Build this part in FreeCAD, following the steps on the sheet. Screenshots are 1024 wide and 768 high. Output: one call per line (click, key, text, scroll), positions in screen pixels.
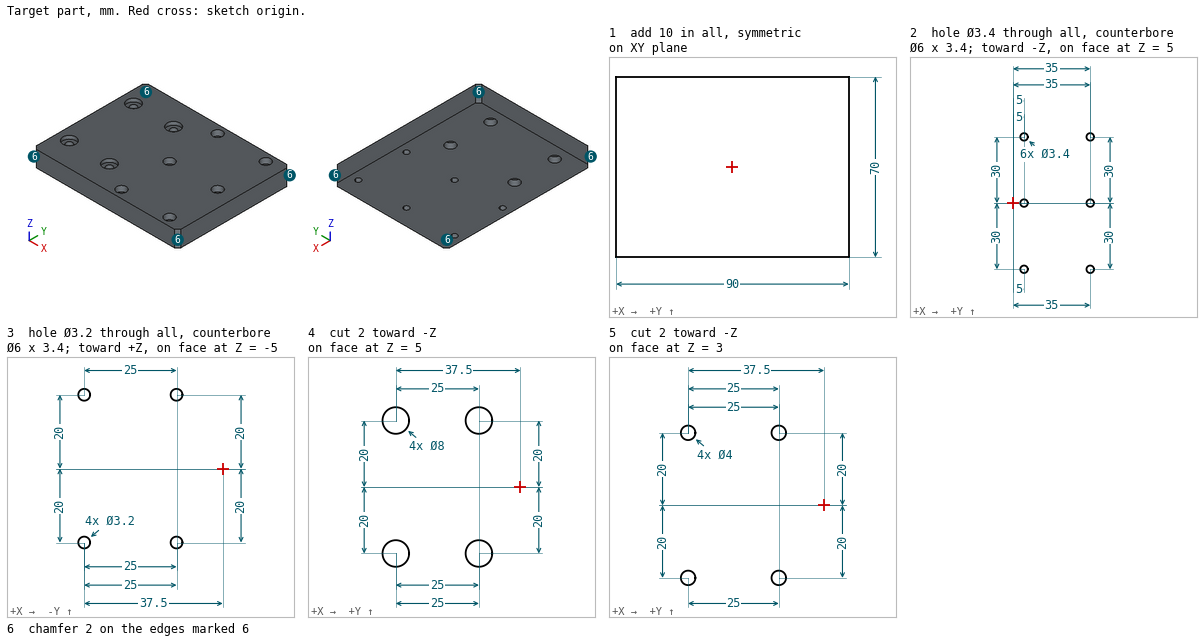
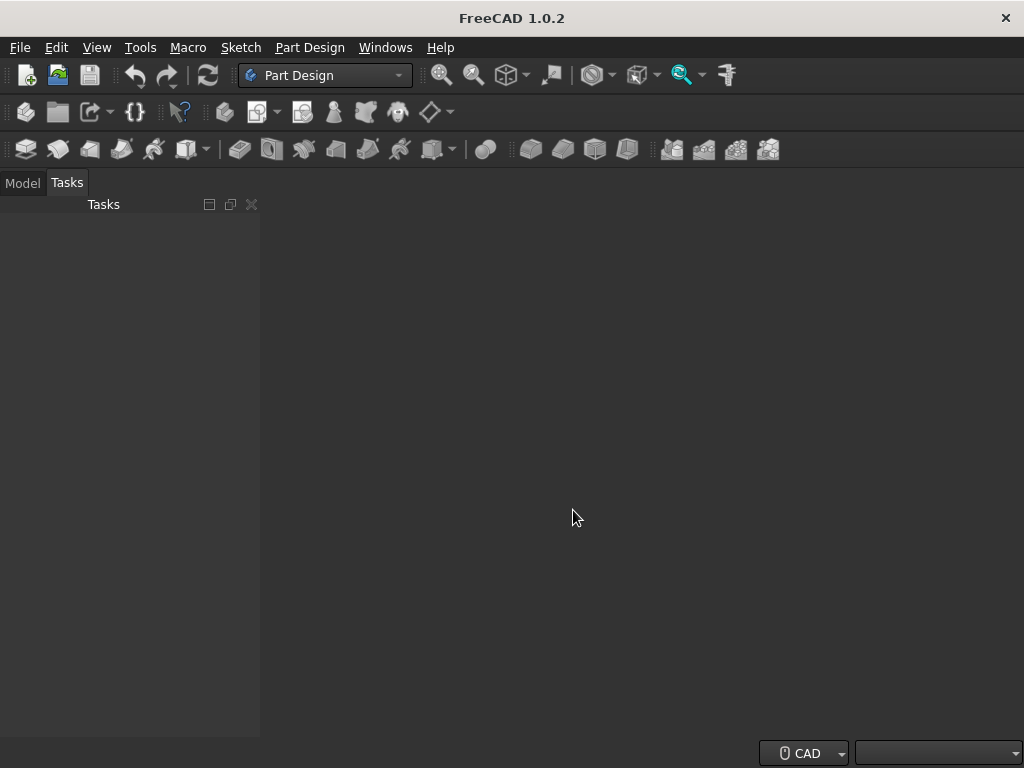
click(26, 76)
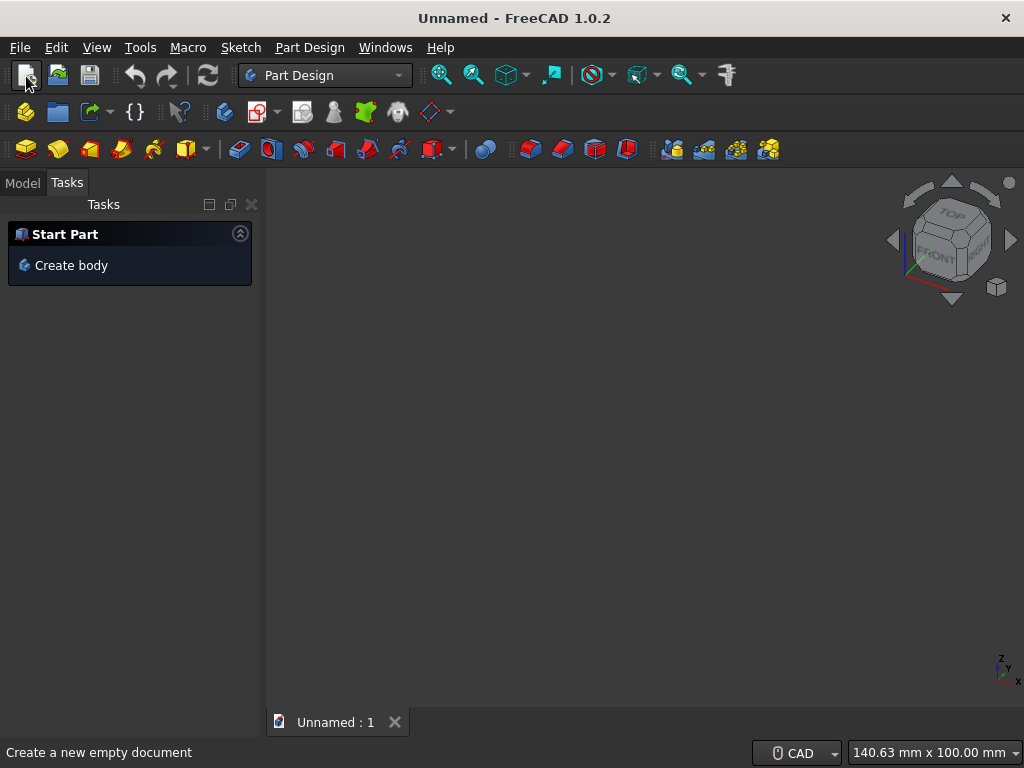
click(258, 112)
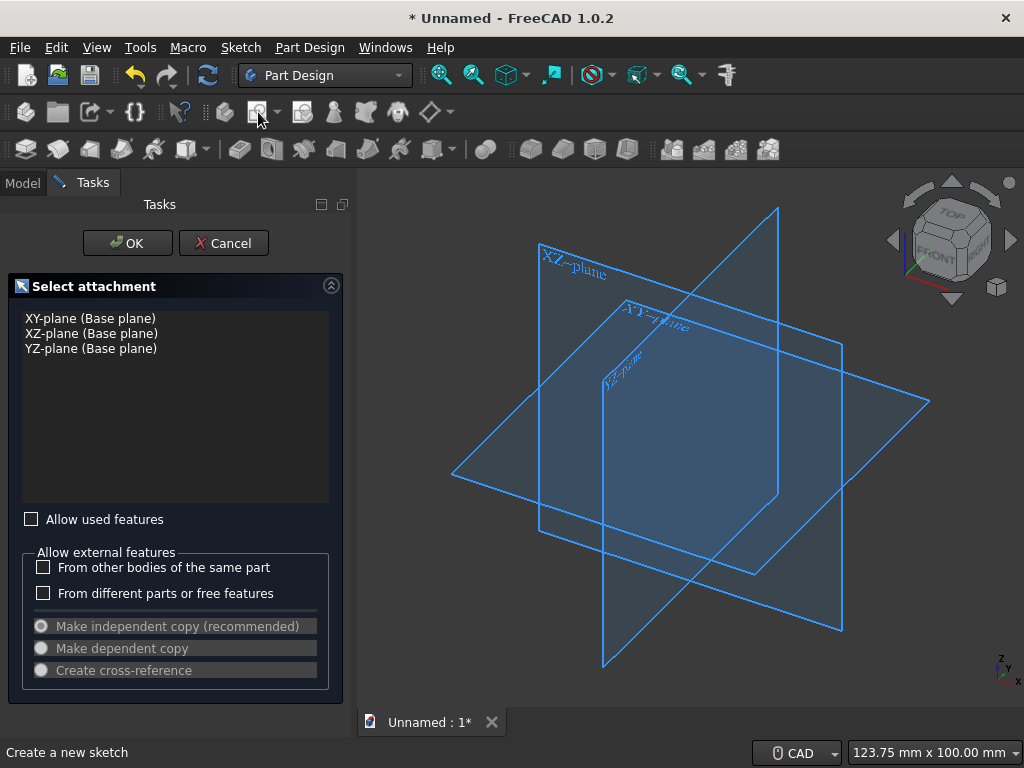
click(82, 318)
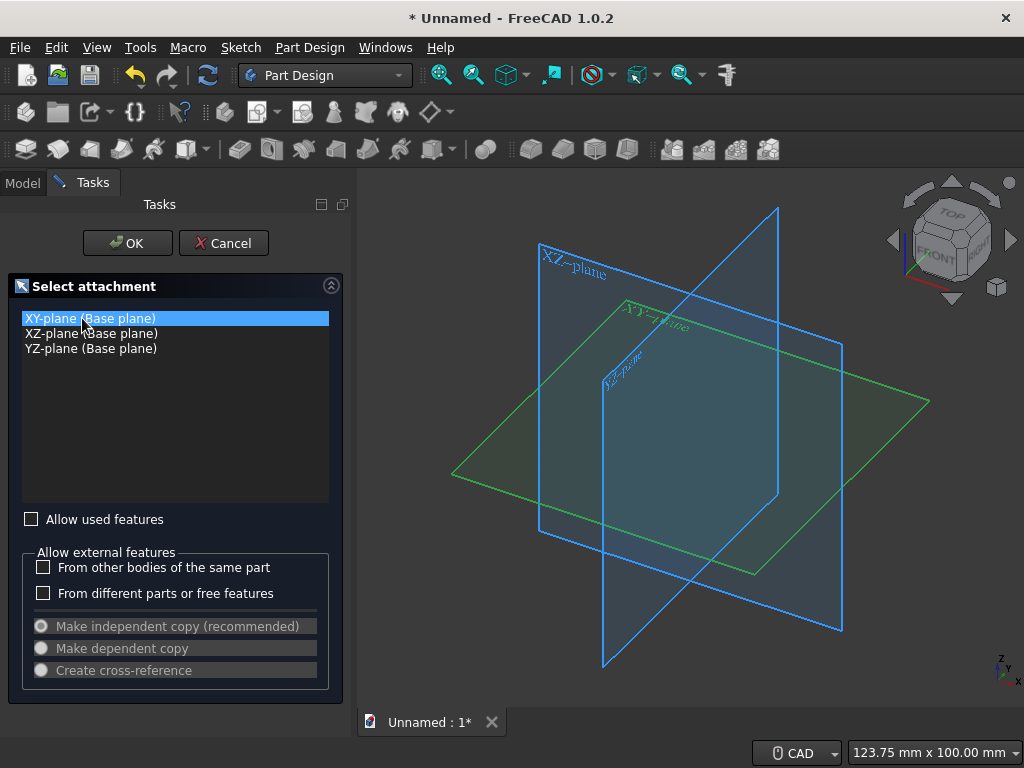
click(128, 243)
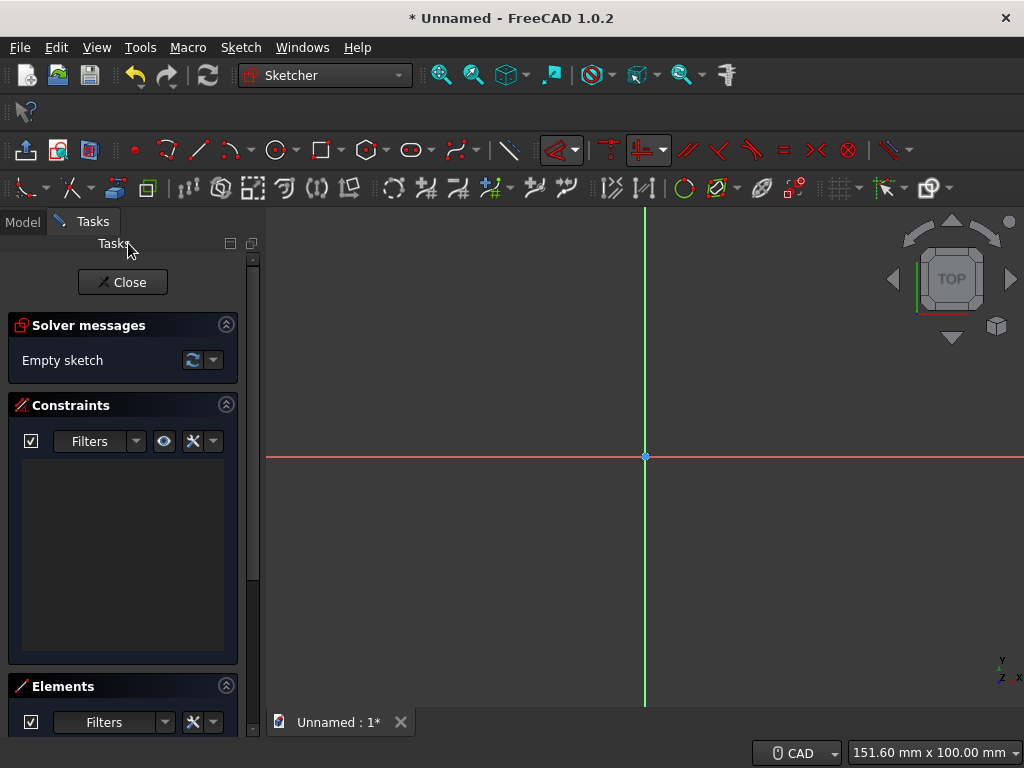
scroll(294, 457, down, 1)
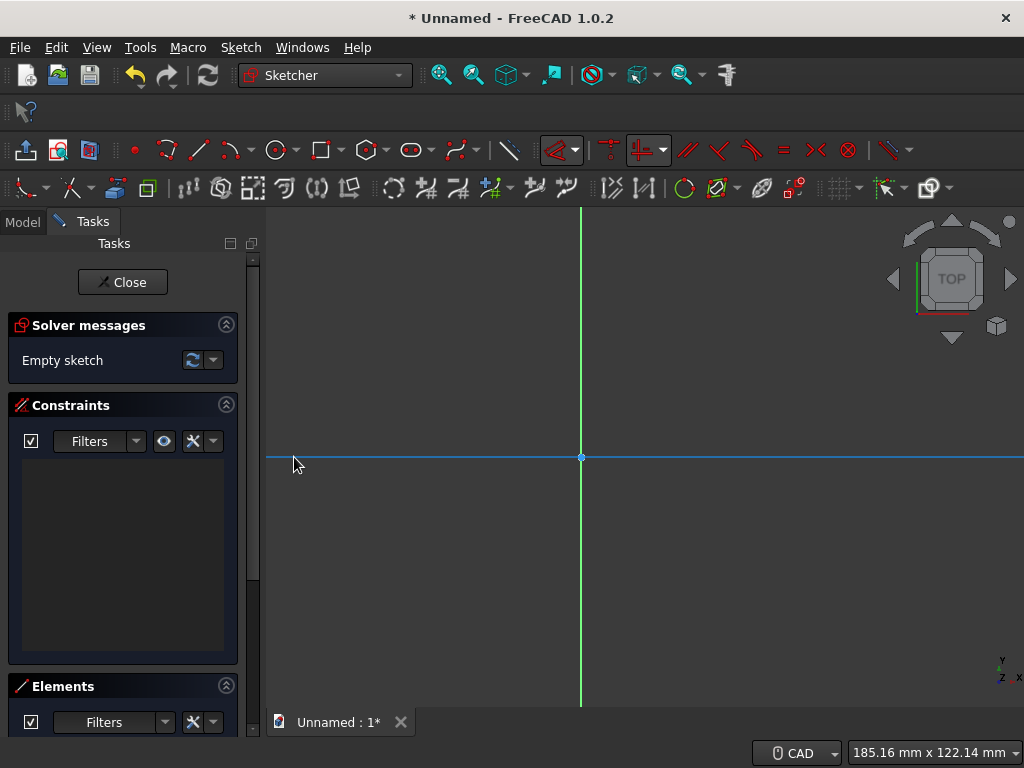
click(344, 150)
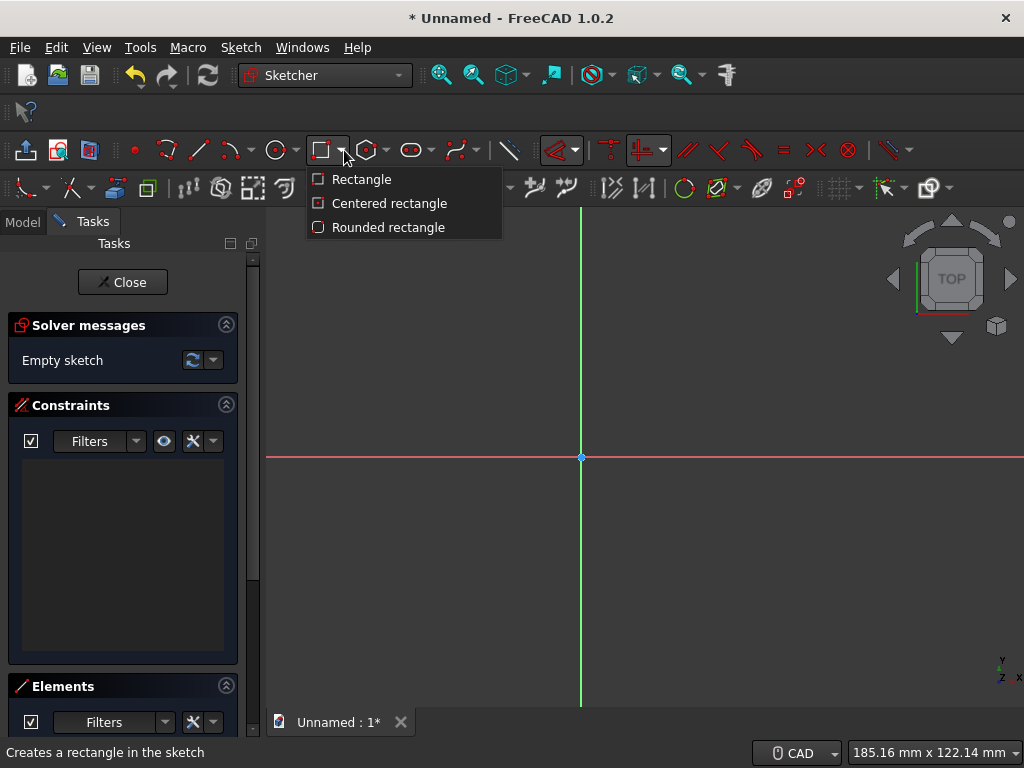
click(404, 203)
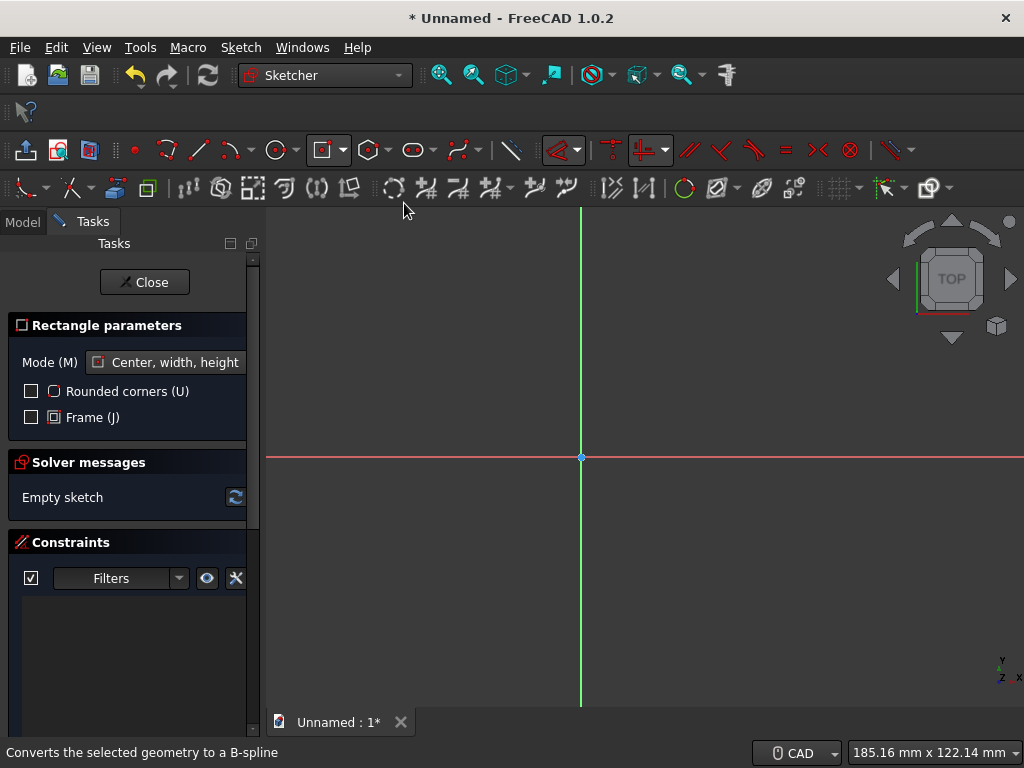
click(581, 457)
click(766, 314)
key(Escape)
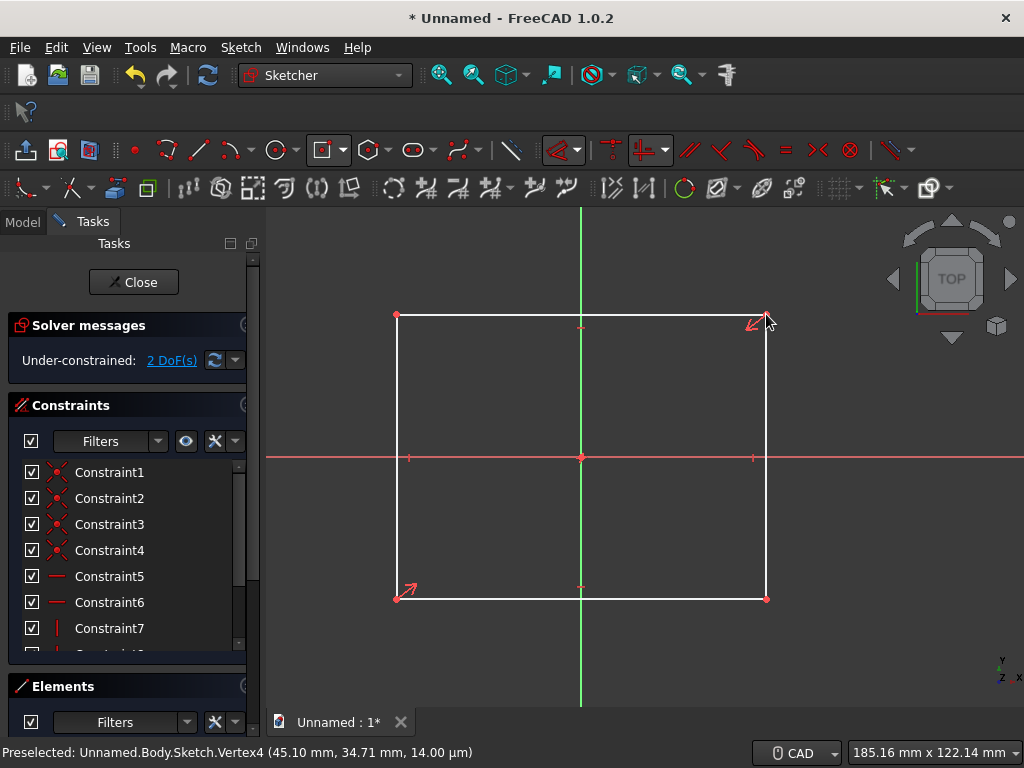
click(558, 150)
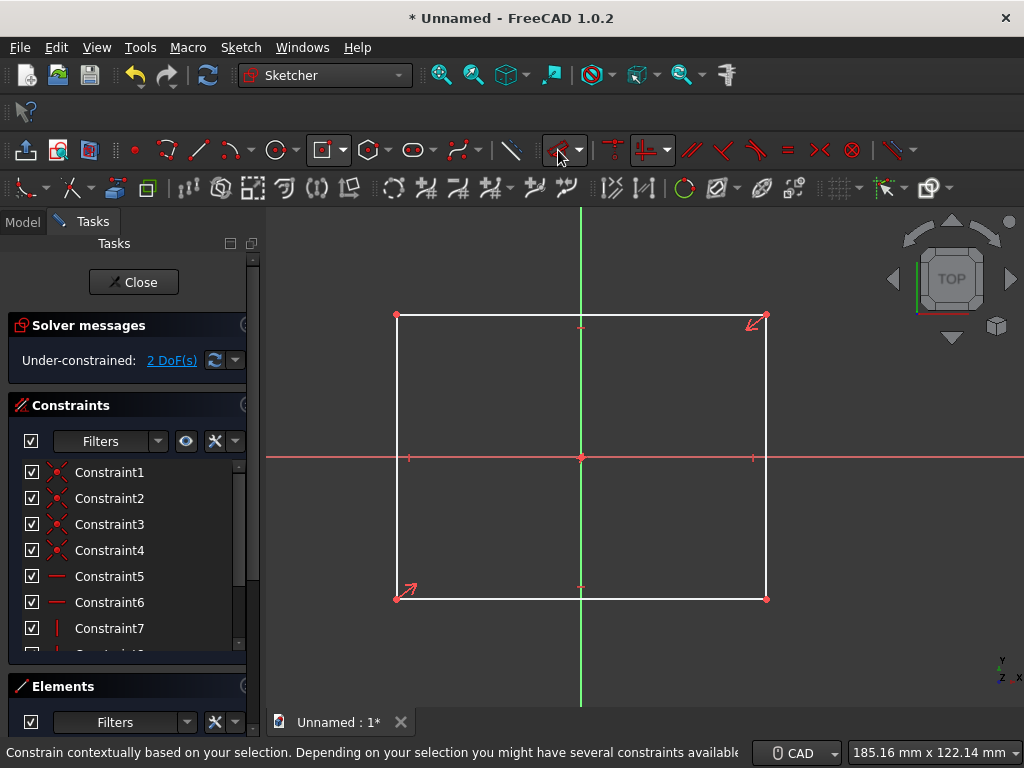
click(508, 599)
click(496, 633)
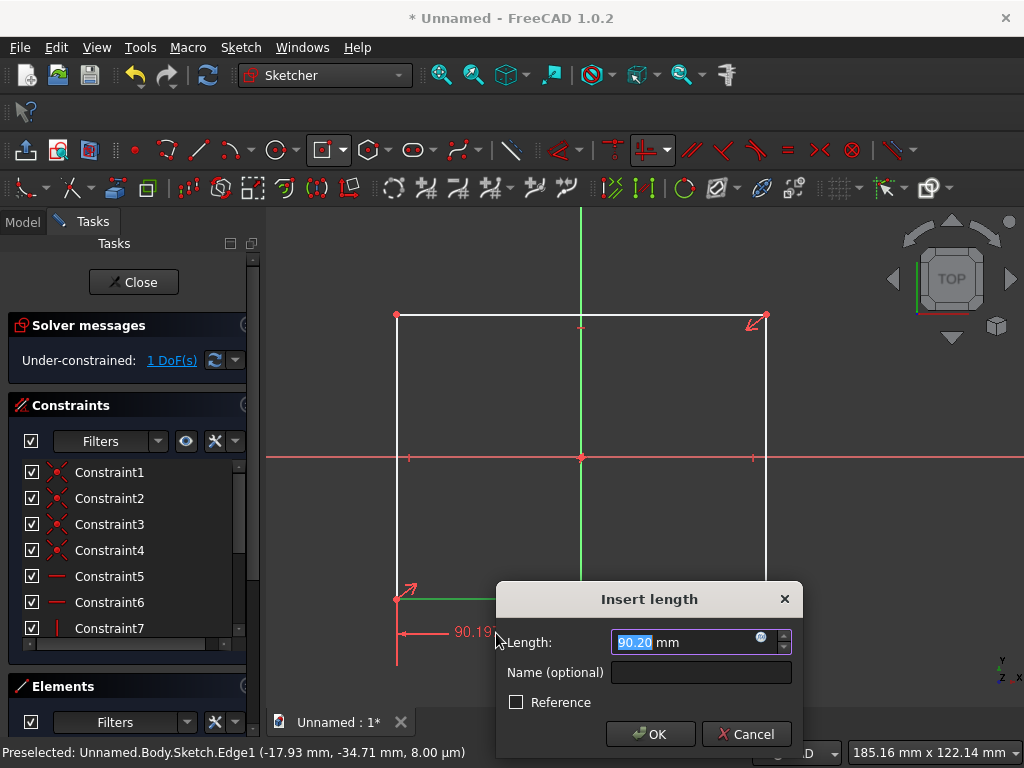
text(90)
key(Return)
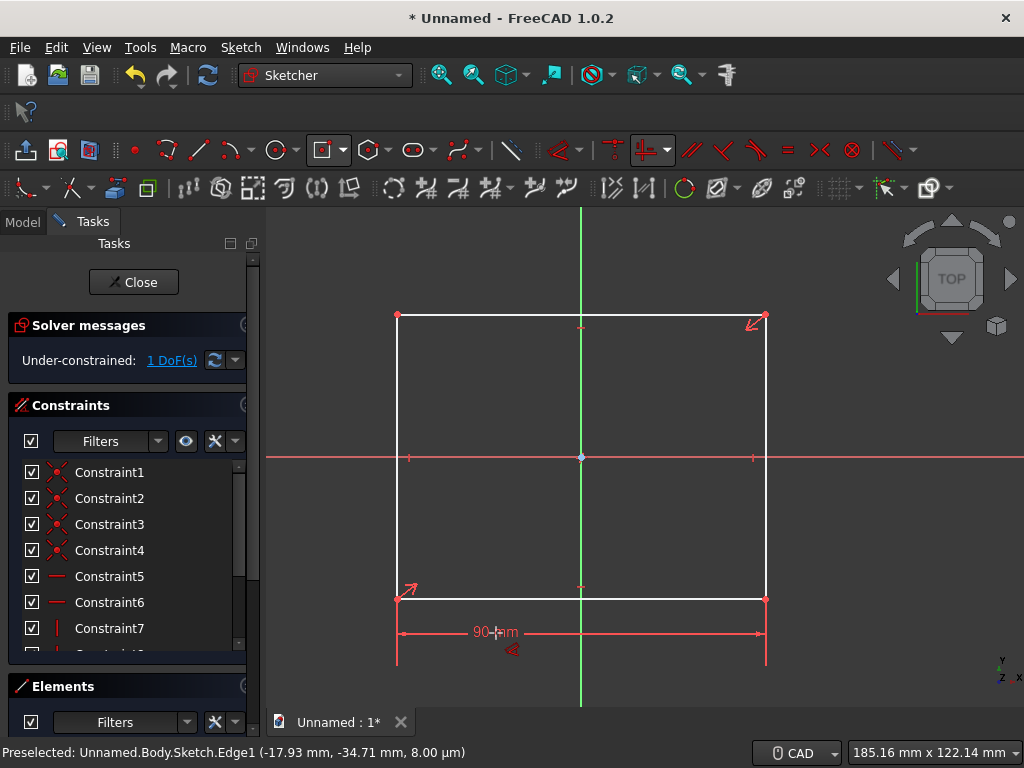
click(766, 514)
click(800, 392)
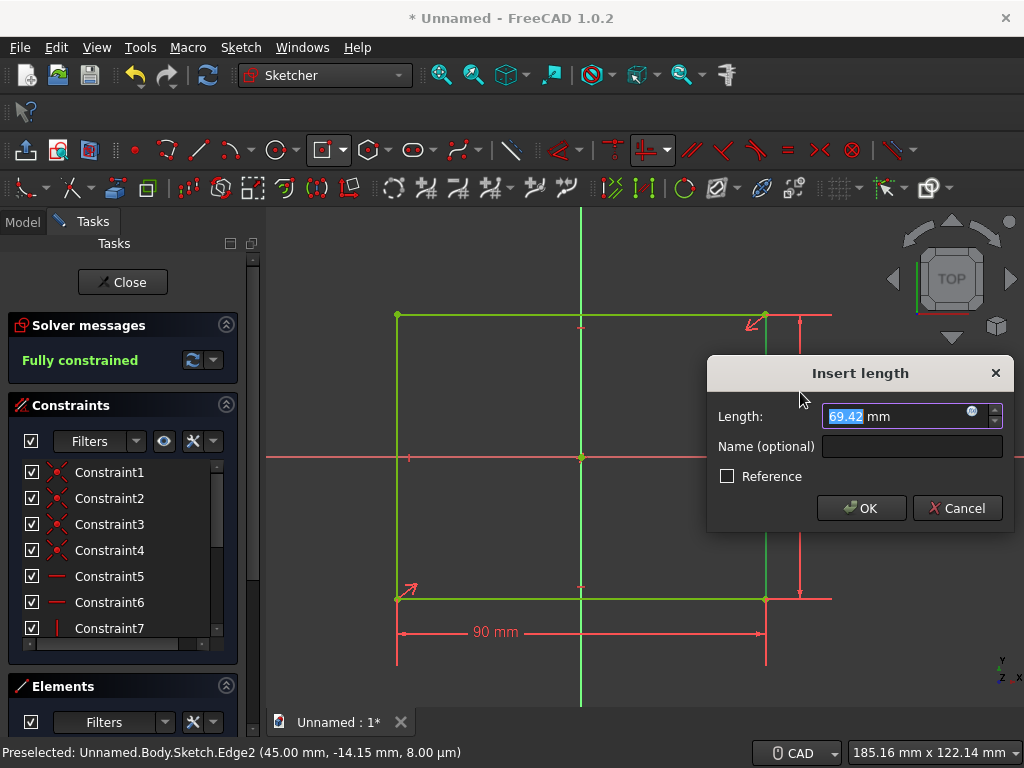
text(70)
key(Return)
key(Escape)